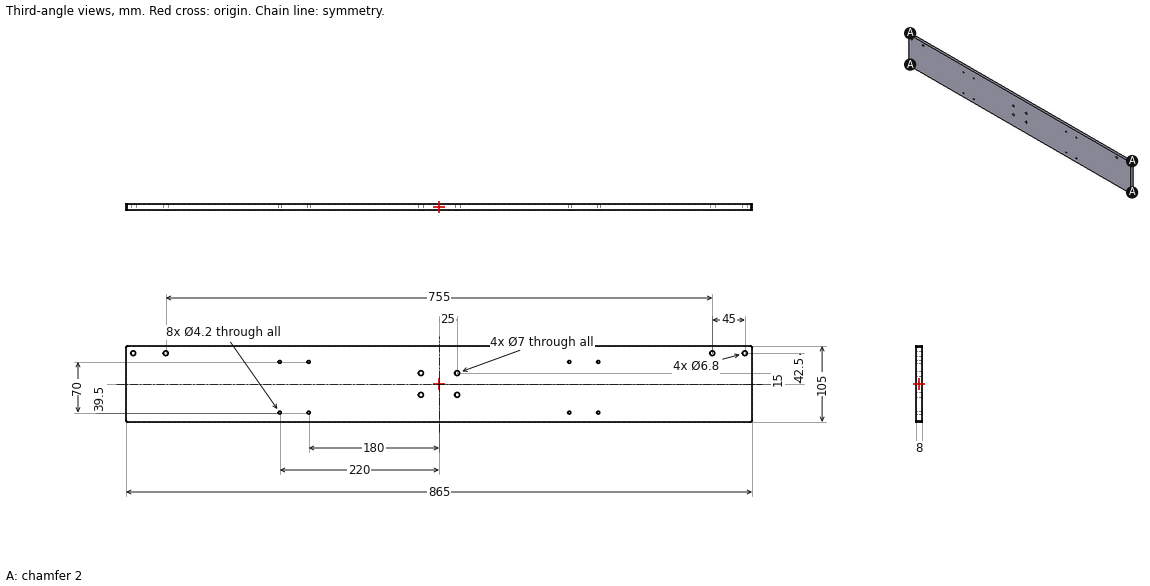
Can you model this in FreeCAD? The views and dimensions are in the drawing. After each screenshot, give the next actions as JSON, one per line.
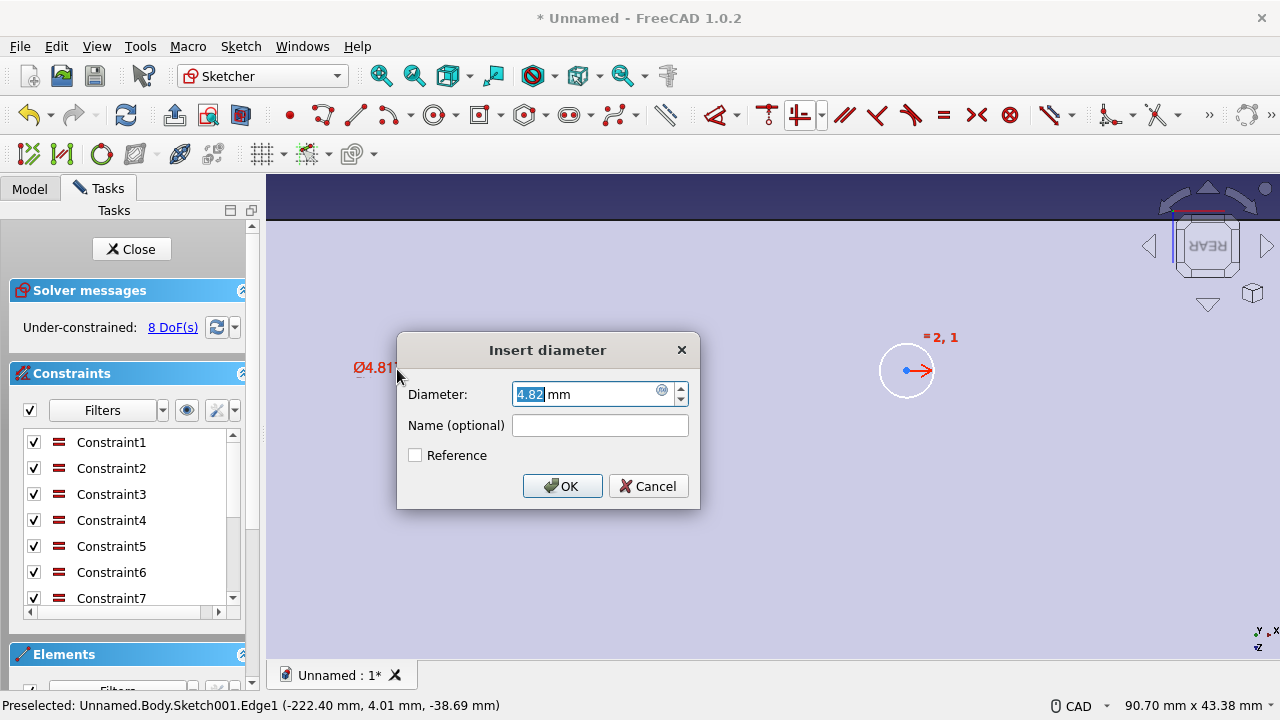
{"action": "type", "text": "4.2"}
{"action": "key", "text": "Return"}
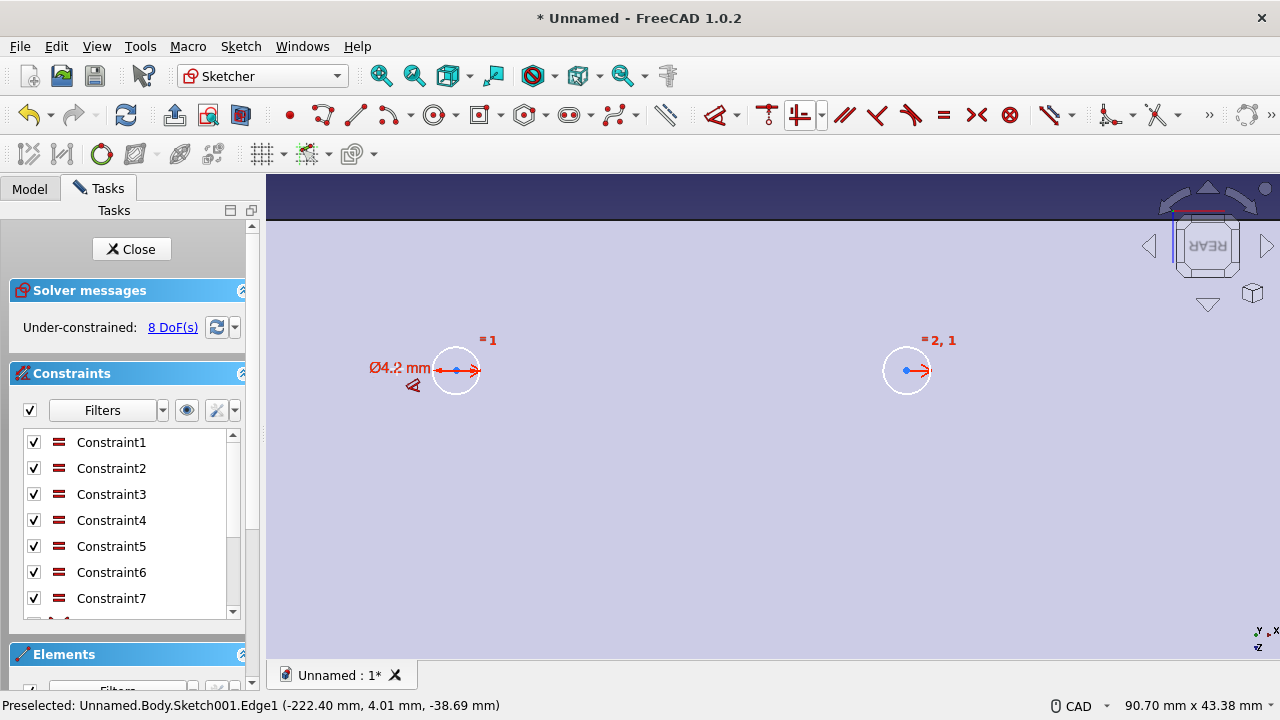
{"action": "scroll", "coordinate": [429, 374], "scroll_direction": "down", "scroll_amount": 11}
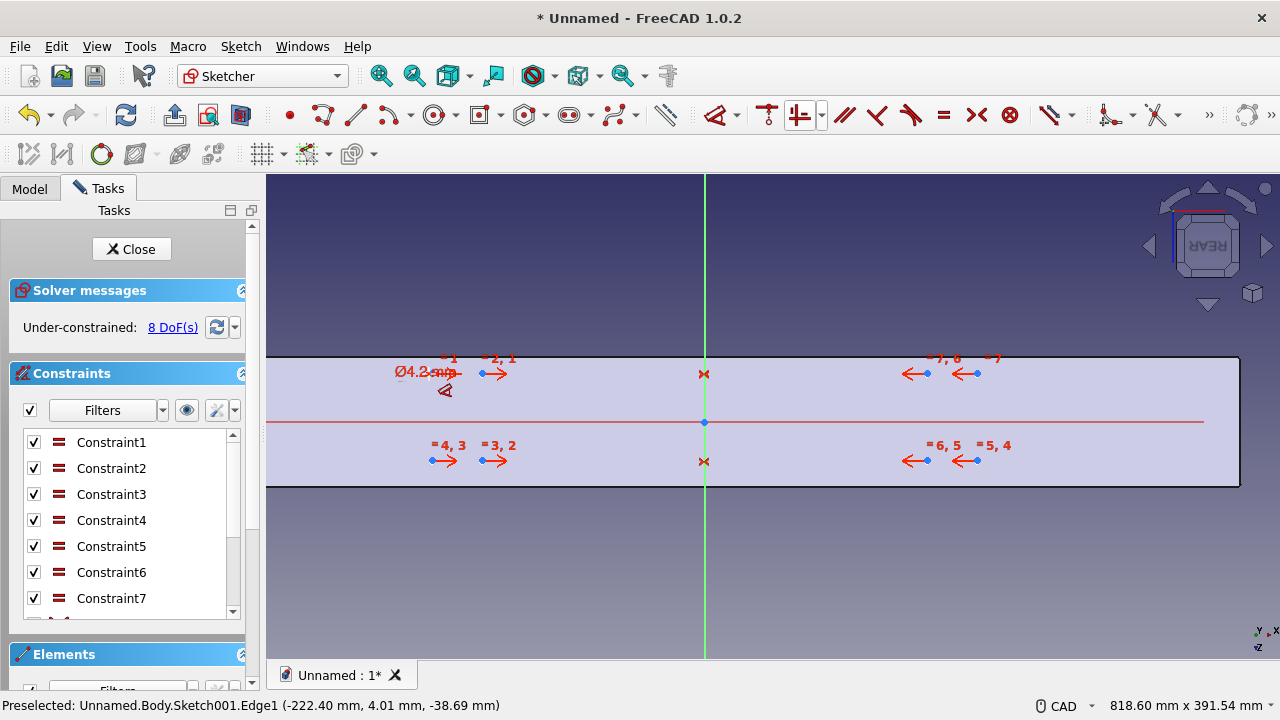
{"action": "left_click", "coordinate": [432, 374]}
{"action": "left_click", "coordinate": [568, 340]}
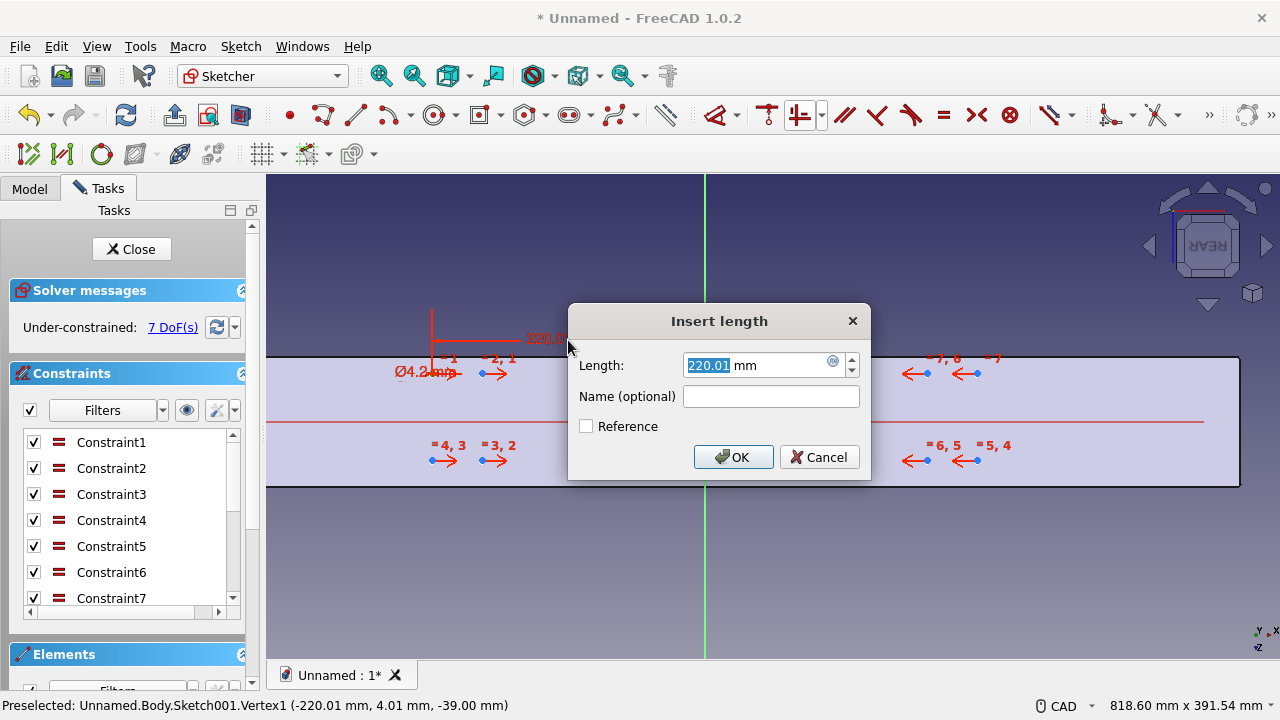
{"action": "type", "text": "220"}
{"action": "key", "text": "Return"}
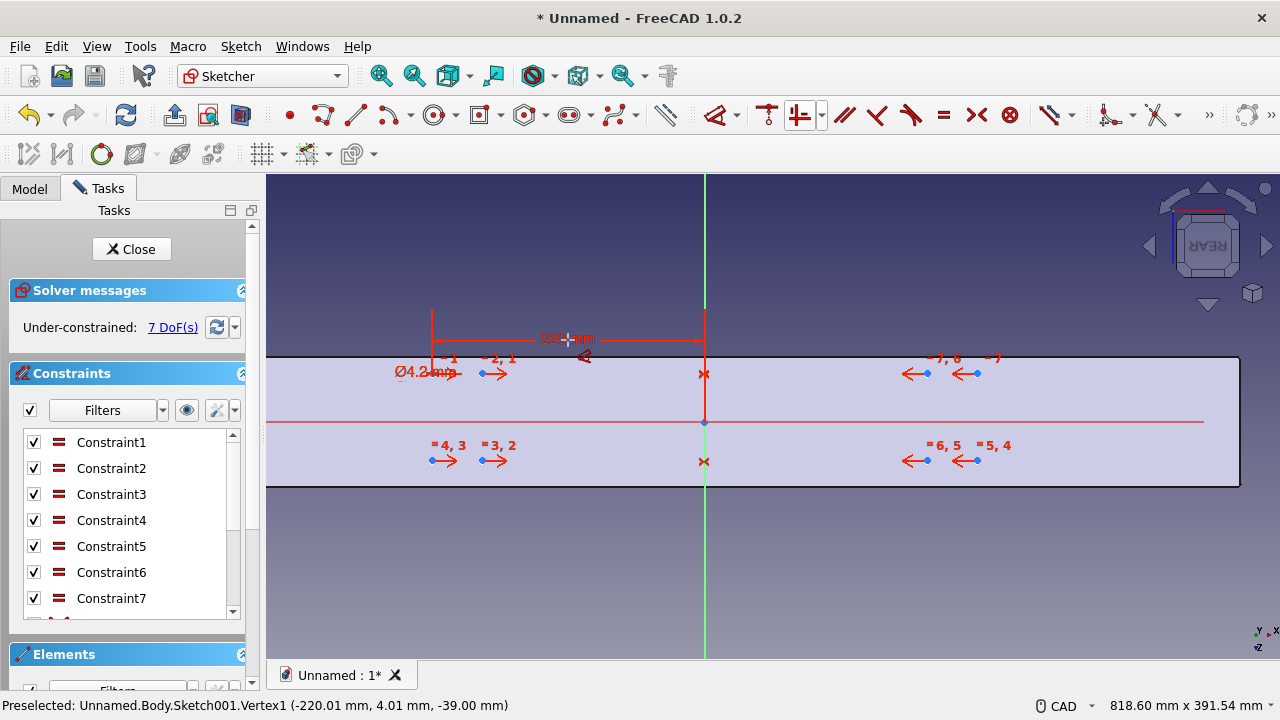
{"action": "left_click", "coordinate": [482, 374]}
{"action": "left_click", "coordinate": [645, 340]}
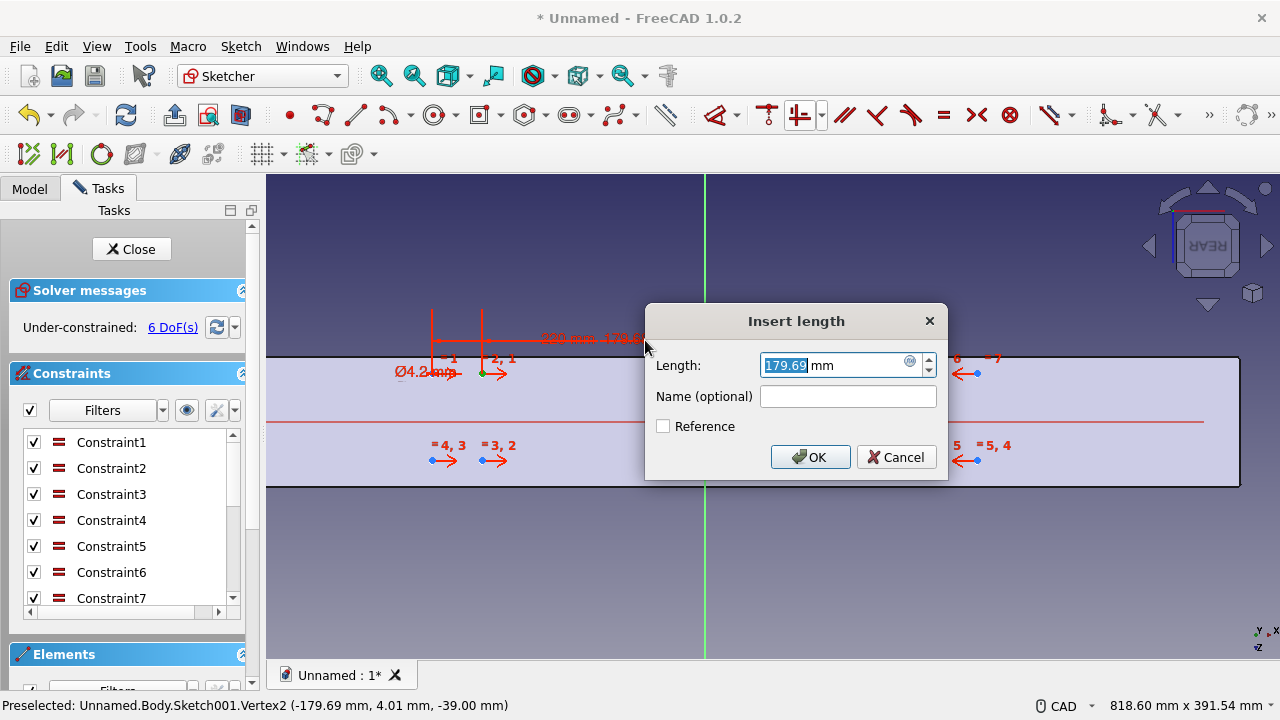
{"action": "type", "text": "180"}
{"action": "key", "text": "Return"}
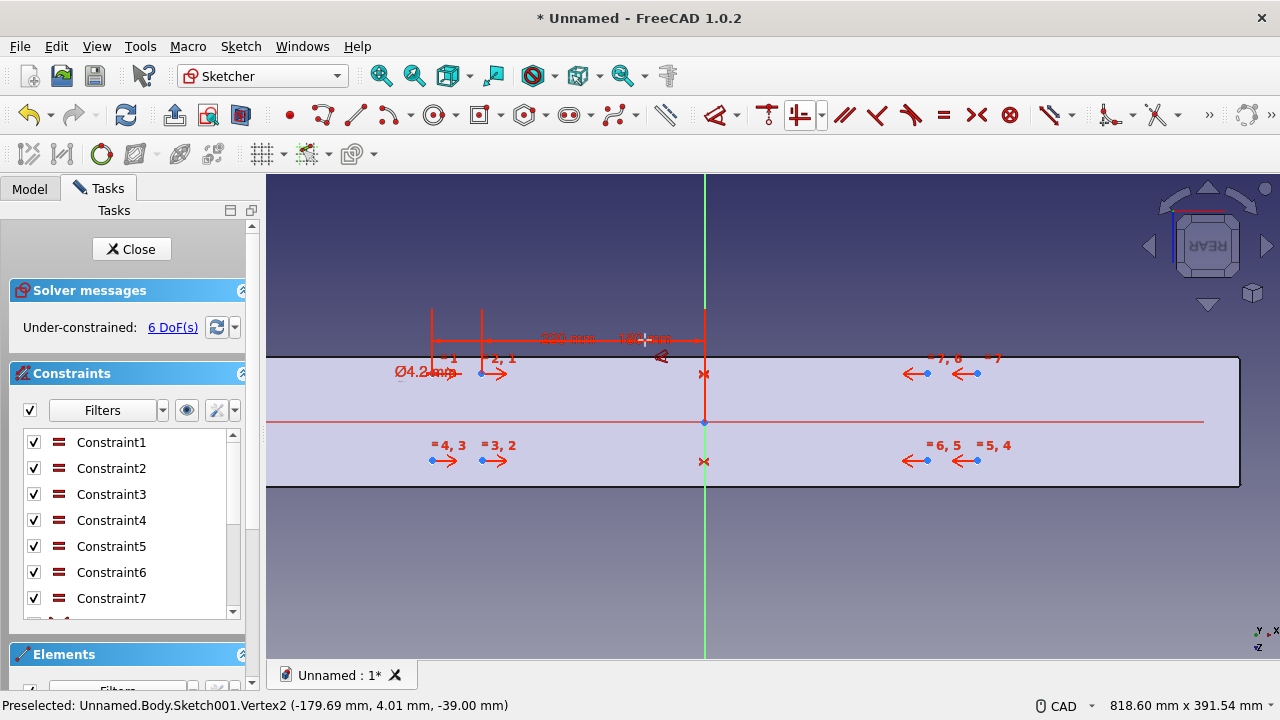
{"action": "left_click", "coordinate": [482, 461]}
{"action": "left_click", "coordinate": [593, 495]}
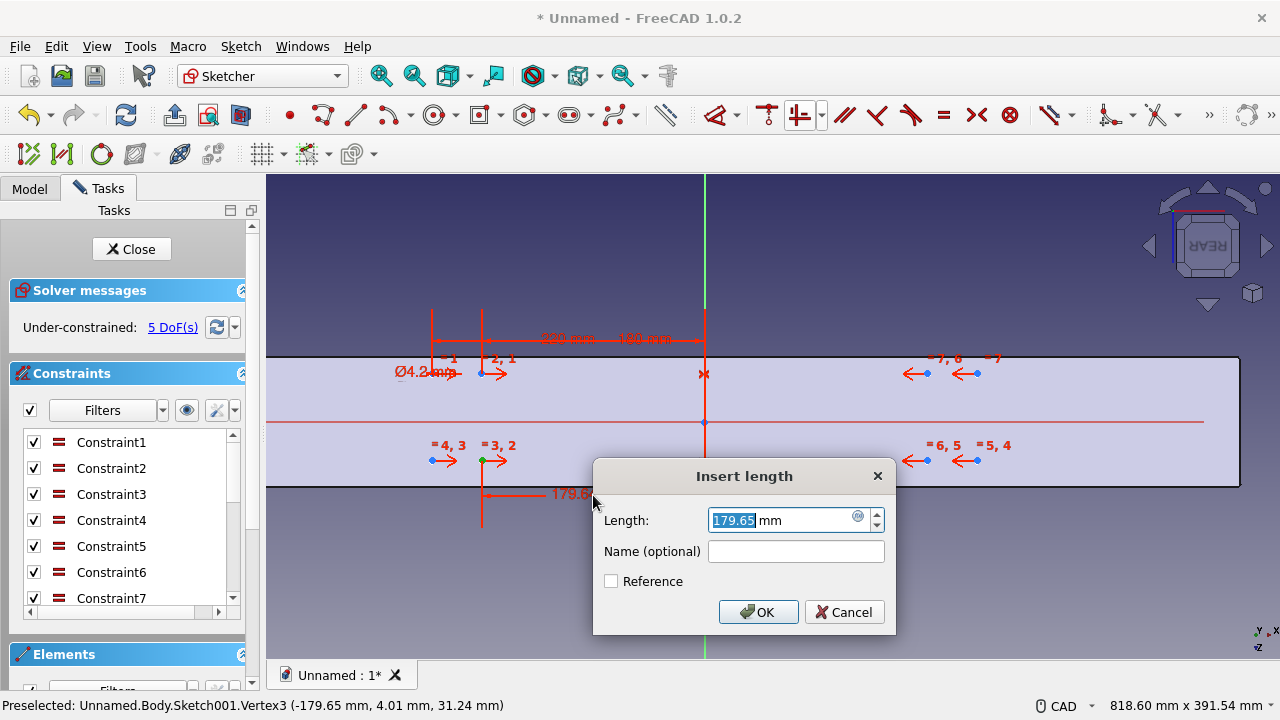
{"action": "type", "text": "180"}
{"action": "key", "text": "Return"}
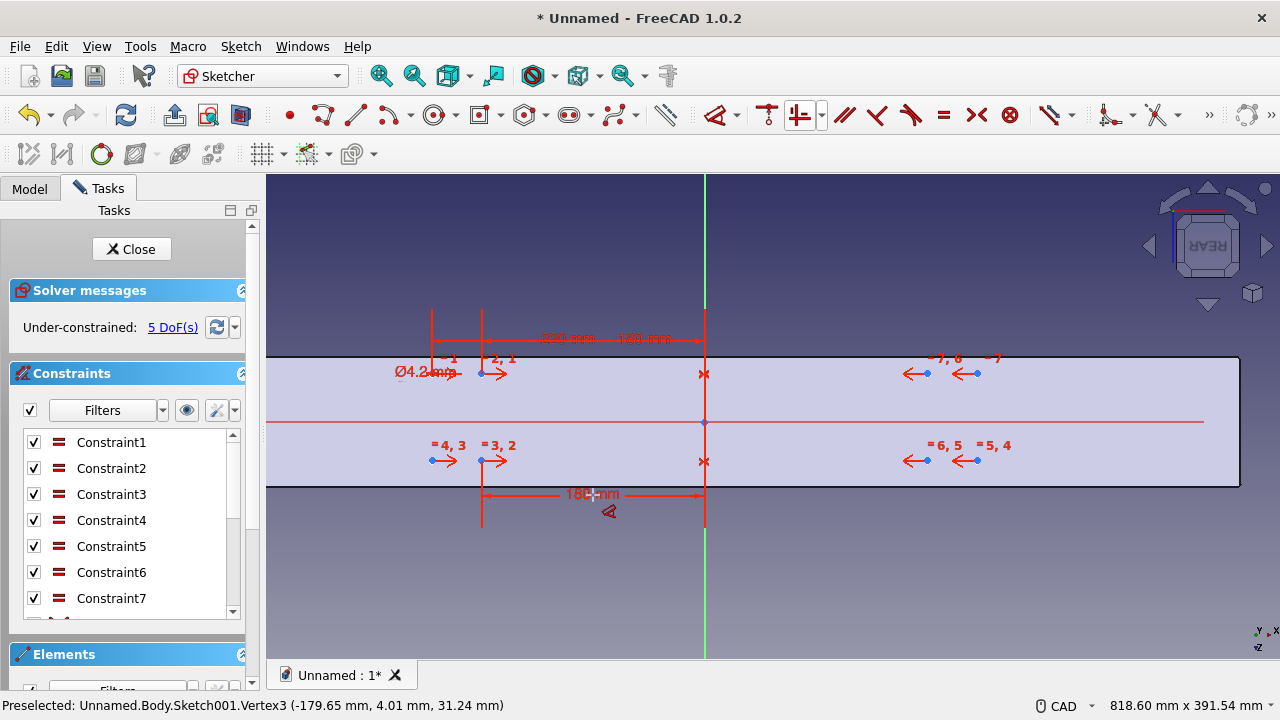
{"action": "left_click", "coordinate": [432, 461]}
{"action": "left_click", "coordinate": [506, 495]}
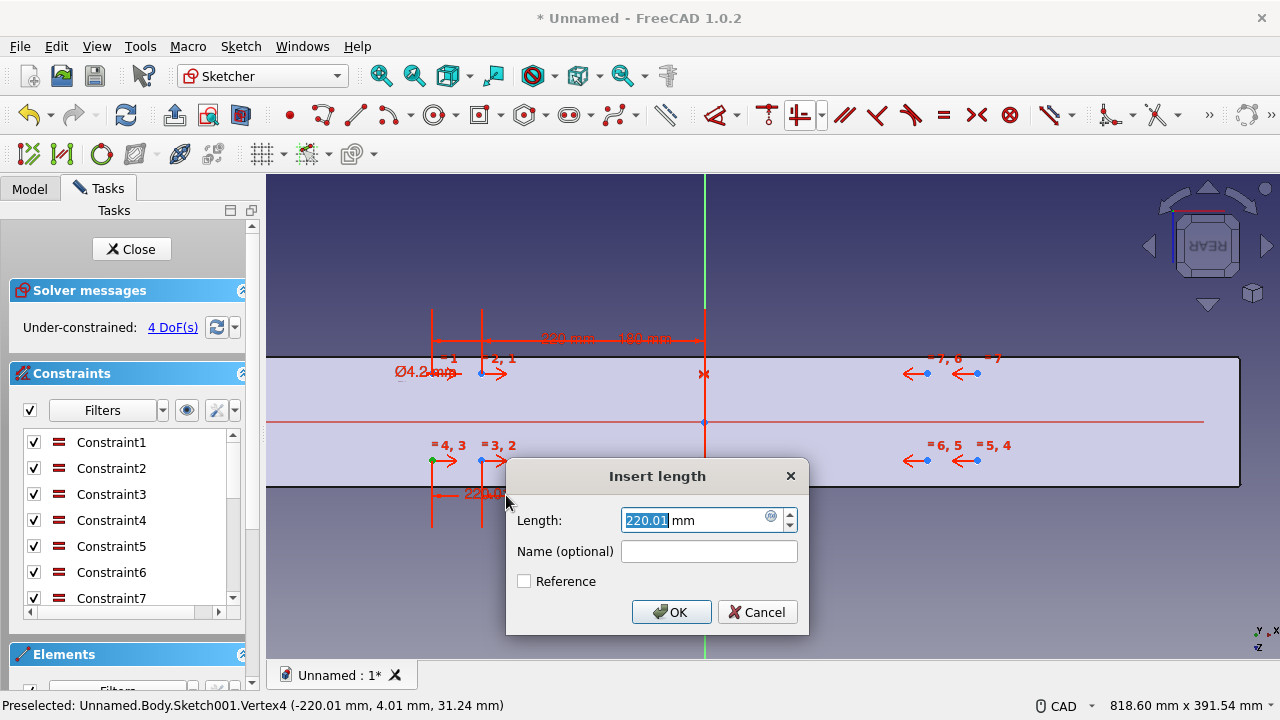
{"action": "type", "text": "220"}
{"action": "key", "text": "Return"}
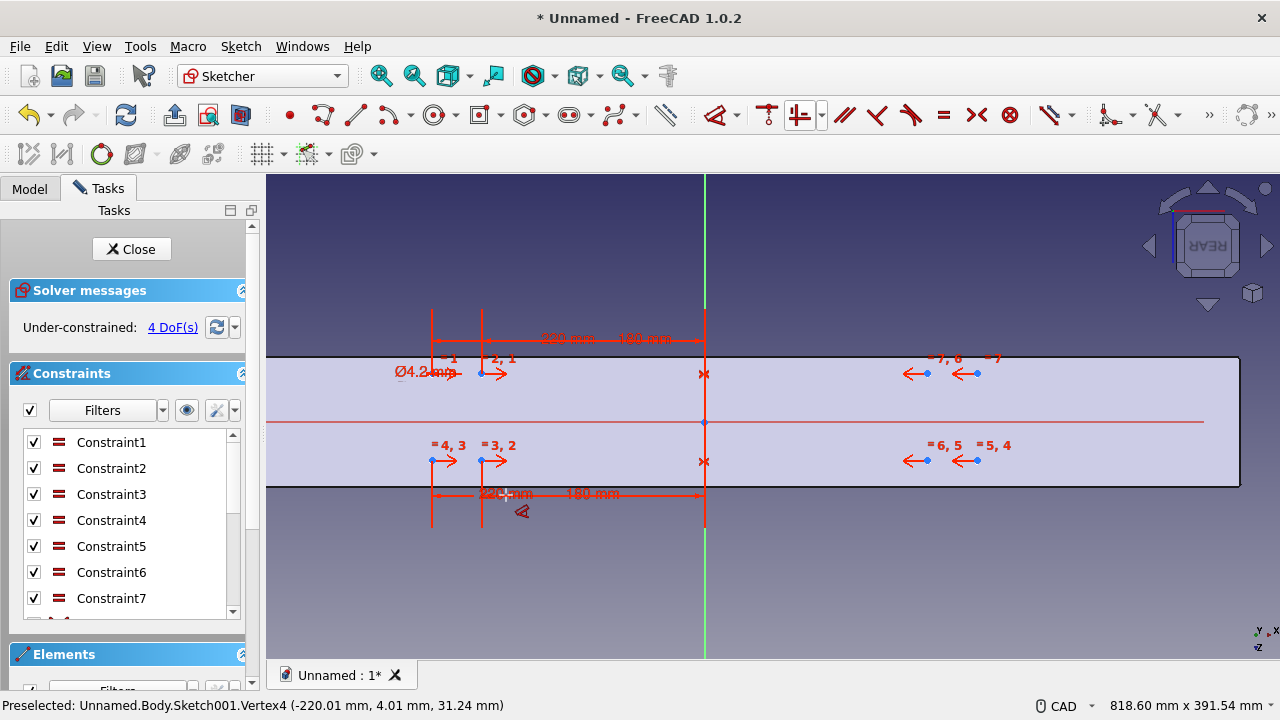
{"action": "left_click", "coordinate": [482, 374]}